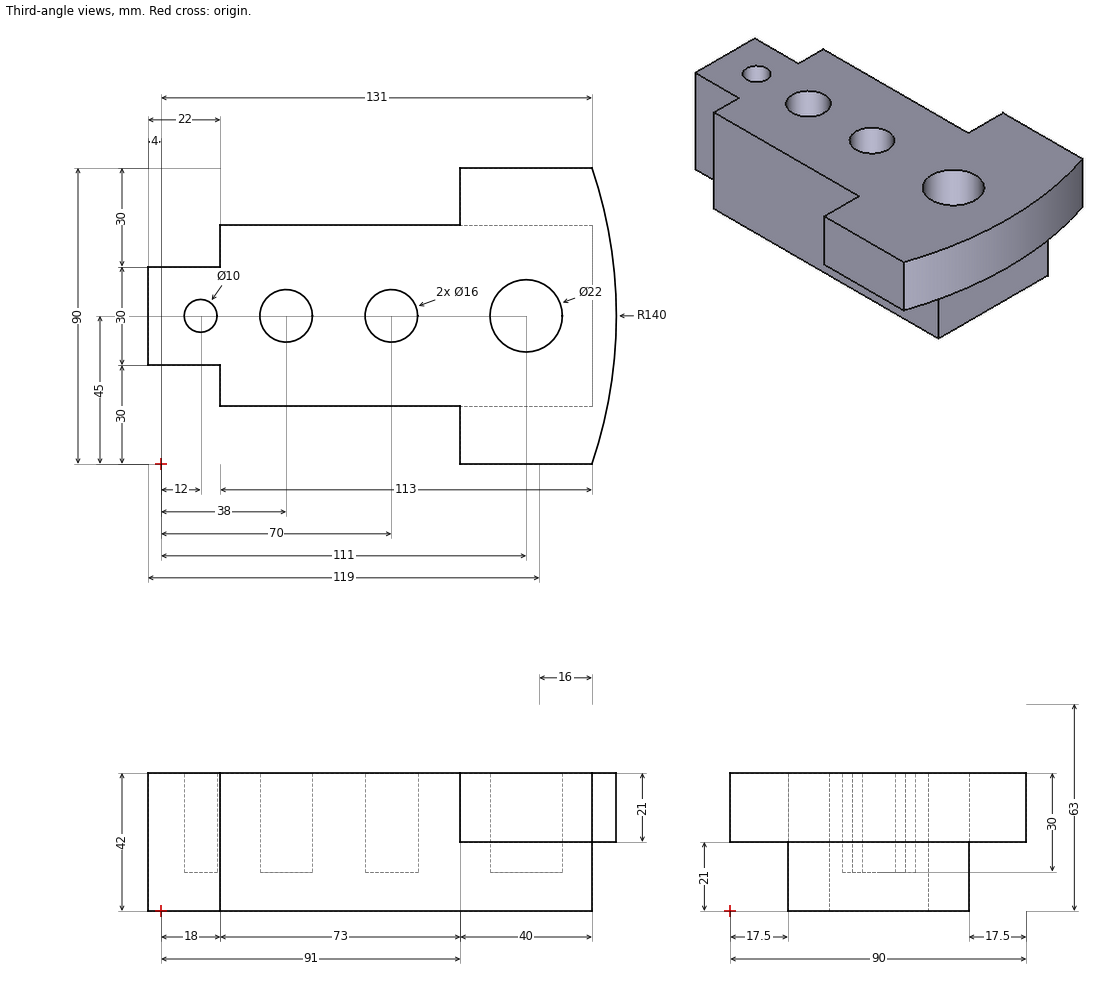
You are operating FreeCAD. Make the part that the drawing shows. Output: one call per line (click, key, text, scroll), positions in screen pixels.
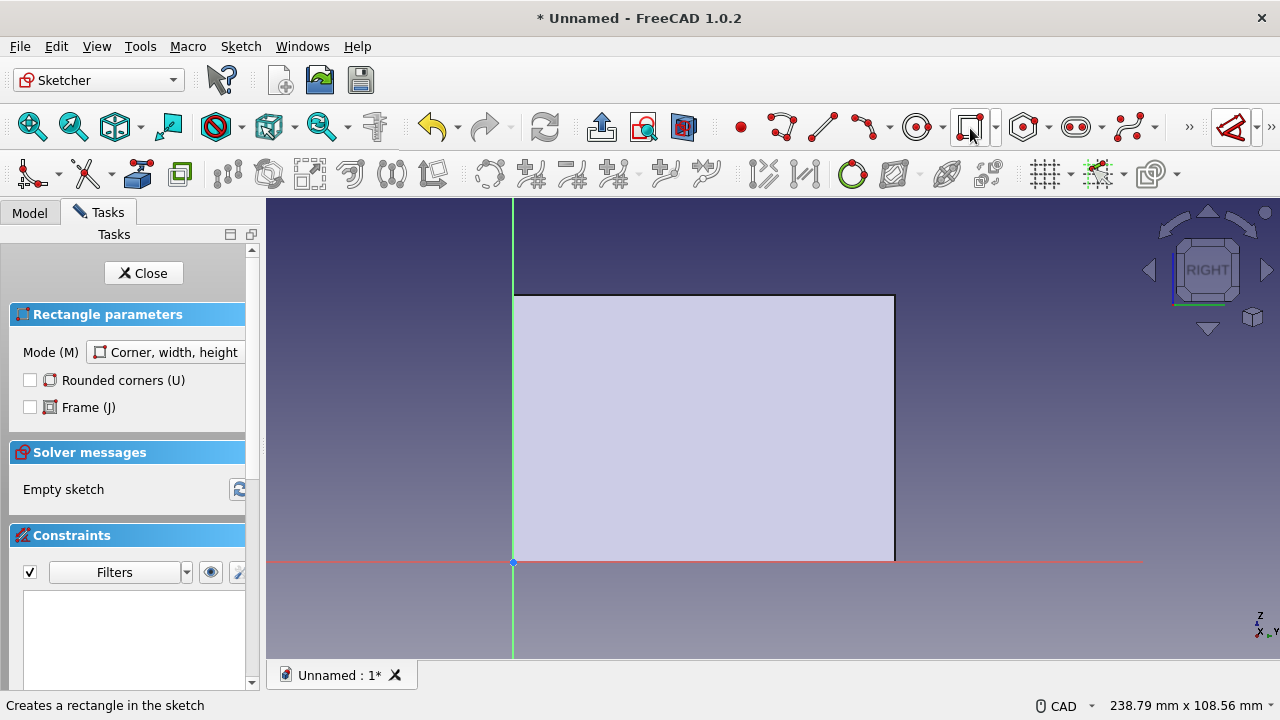
click(513, 562)
move(895, 295)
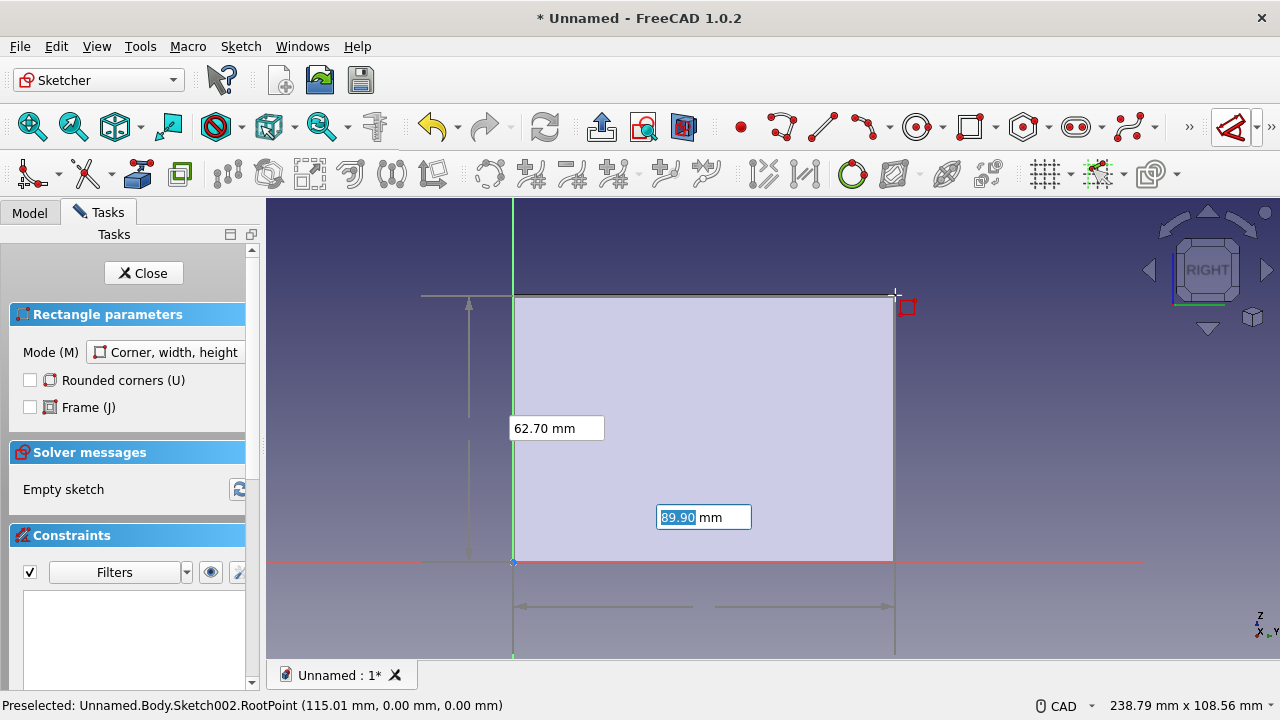
text(90)
key(Tab)
text(63)
key(Return)
key(Escape)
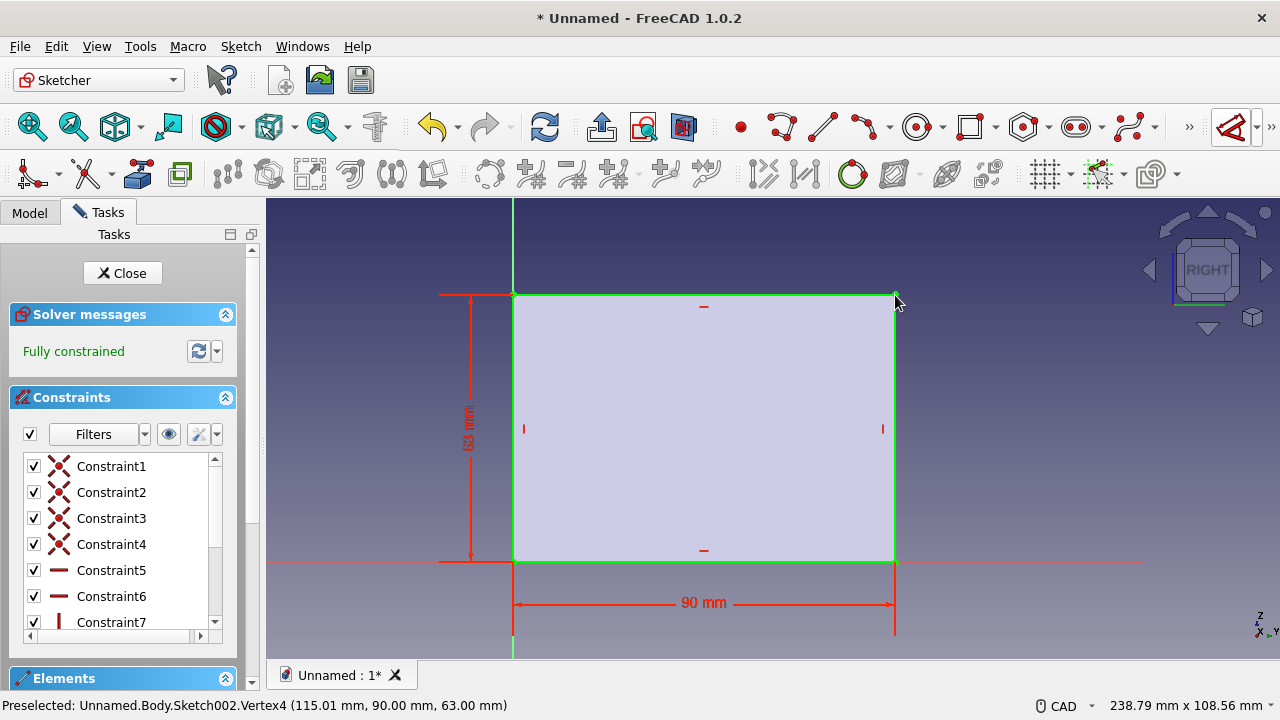
click(123, 273)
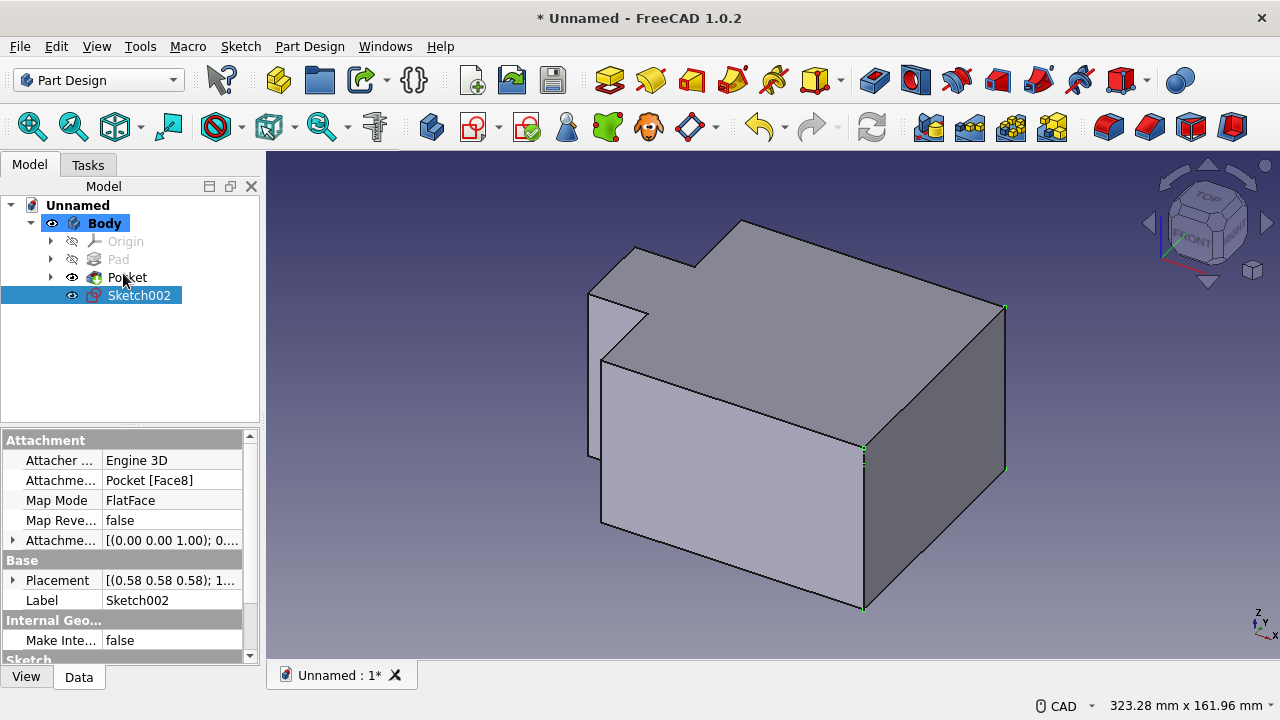
click(610, 80)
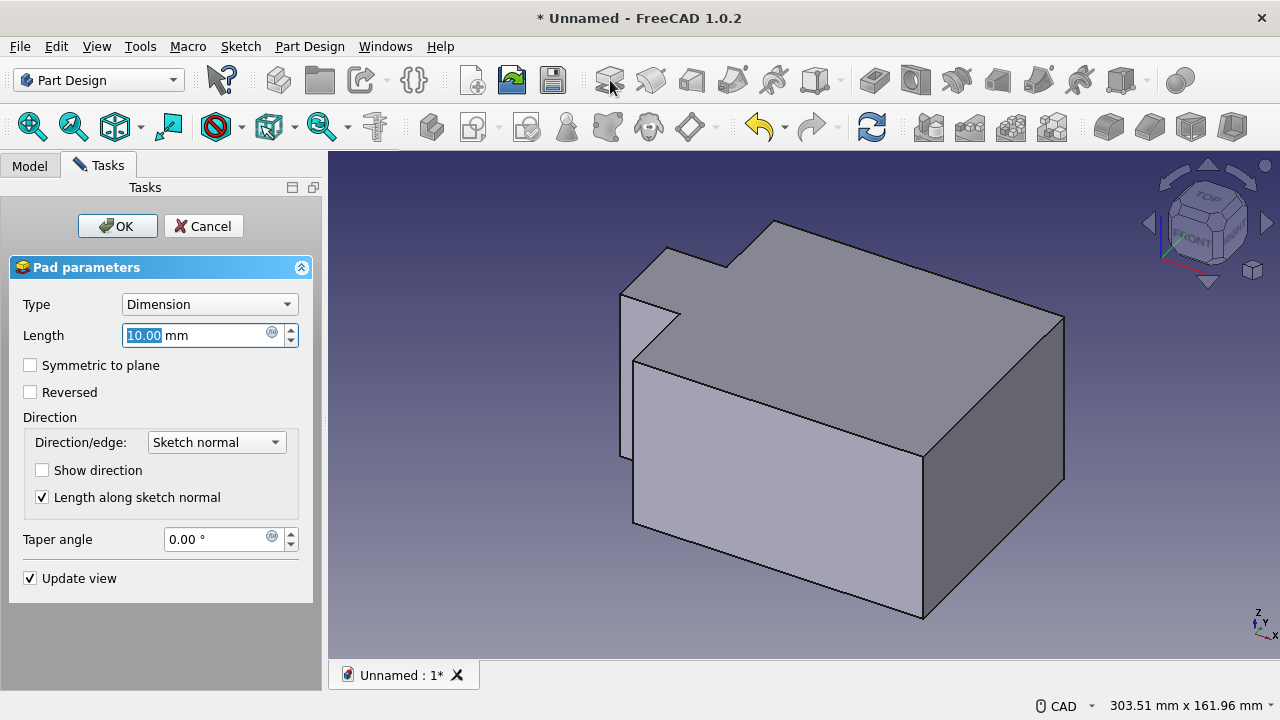
text(16)
key(Tab)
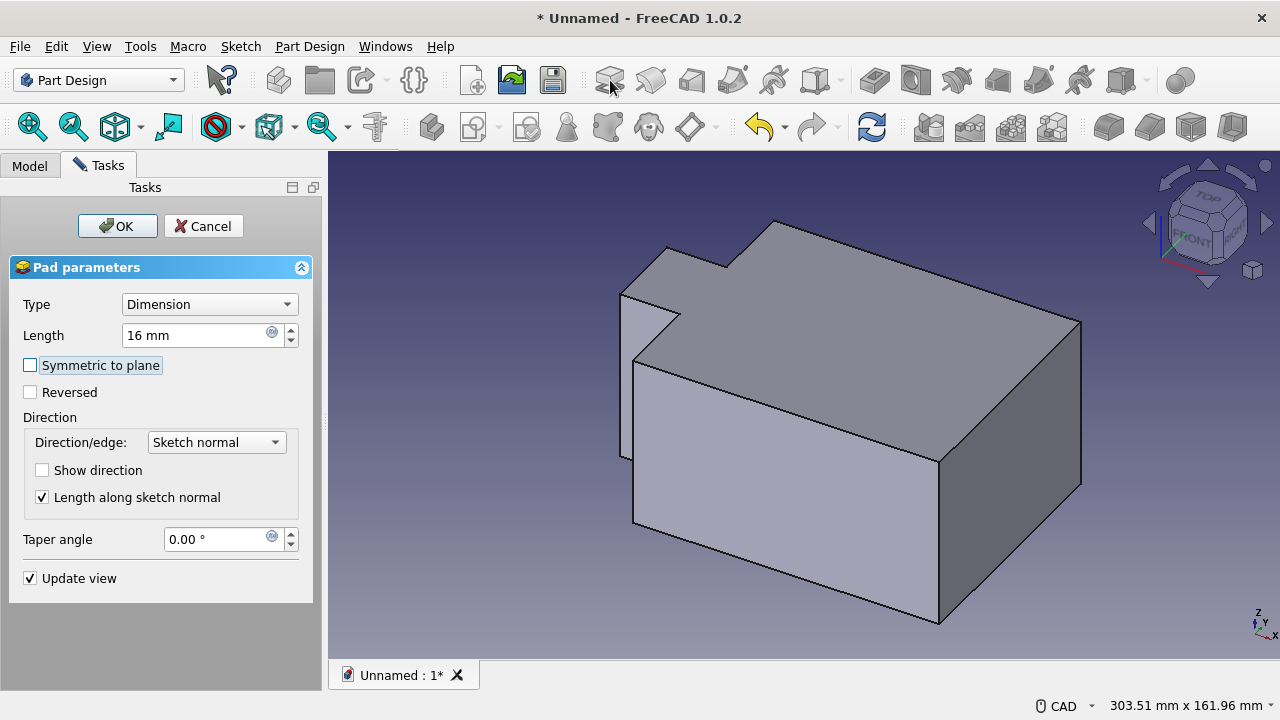
click(118, 226)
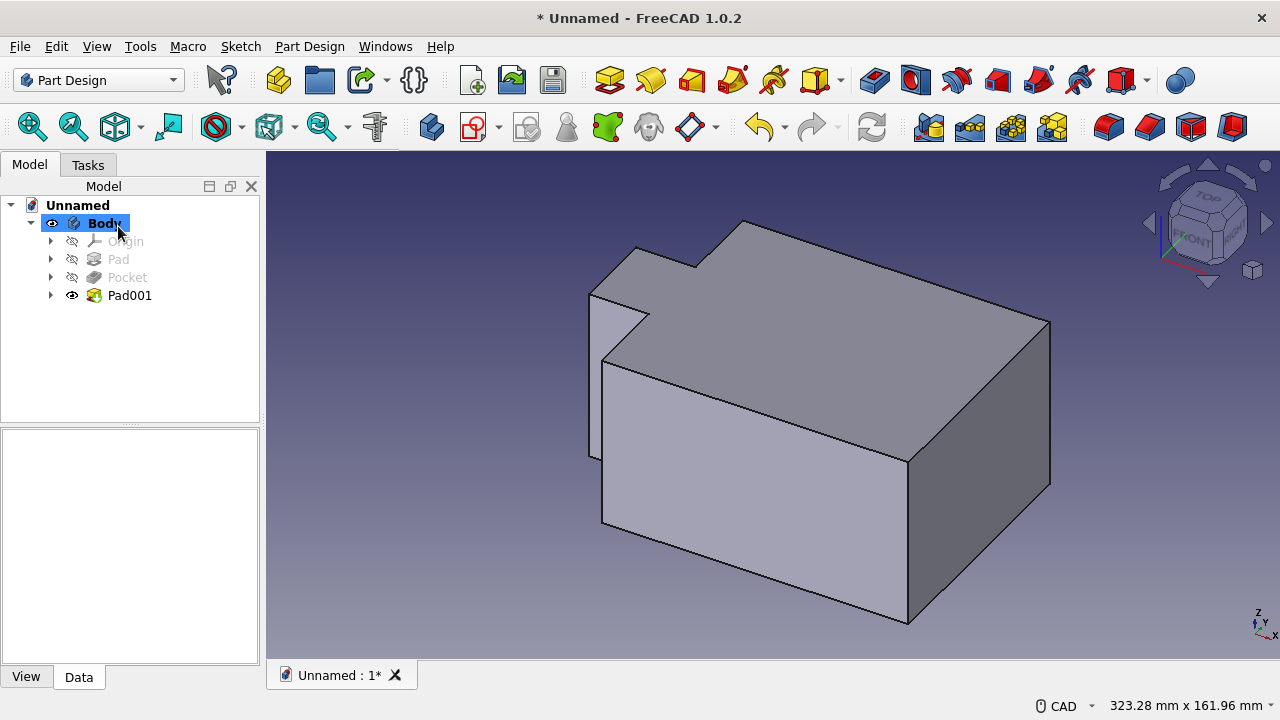
click(848, 348)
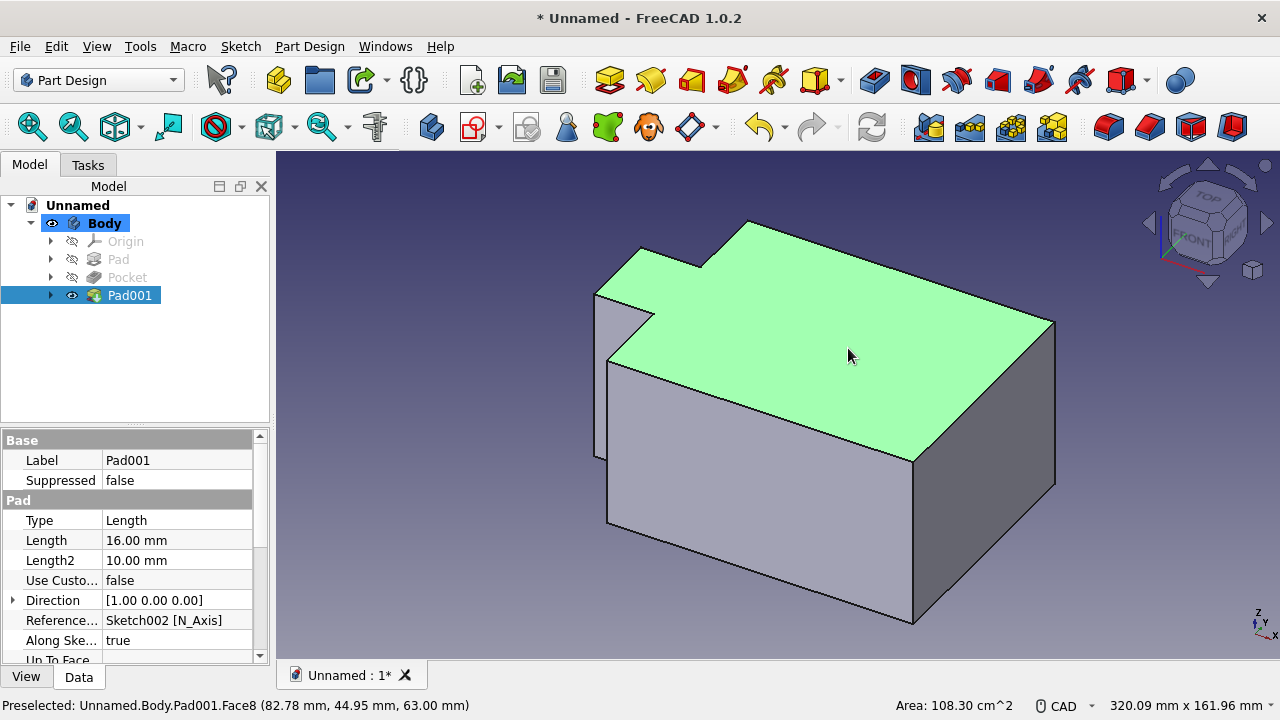
click(472, 128)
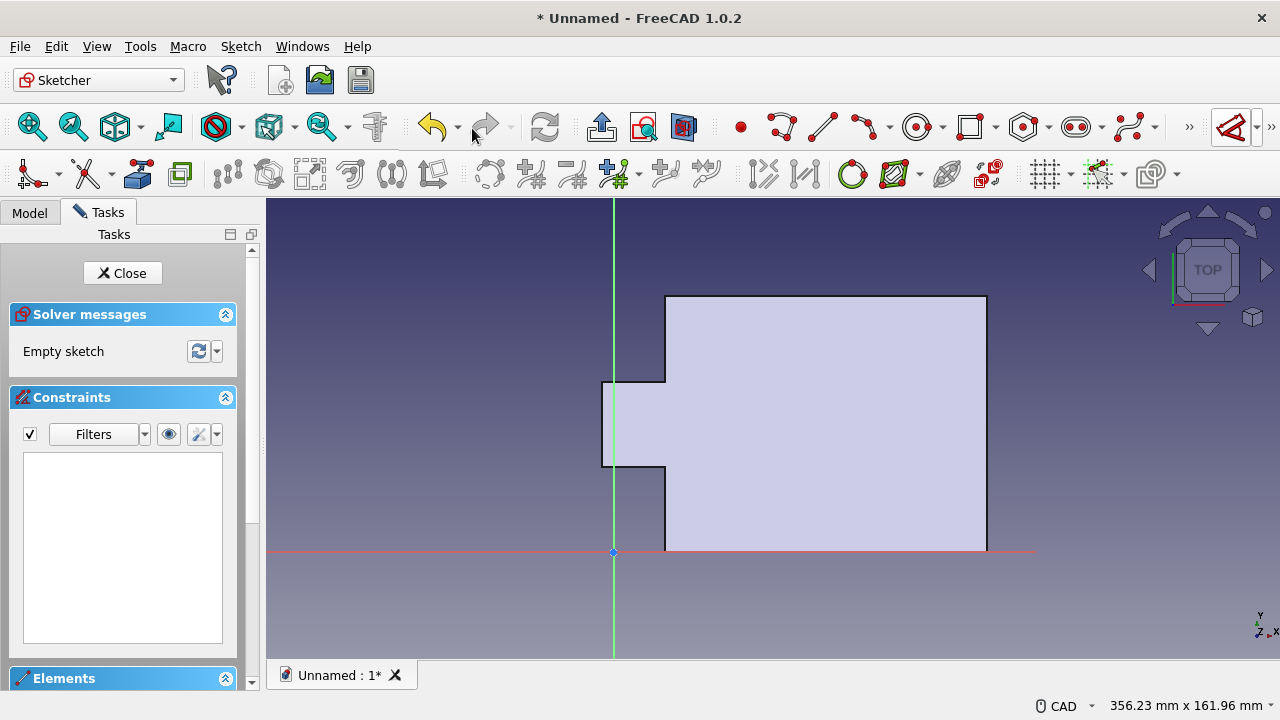
click(782, 128)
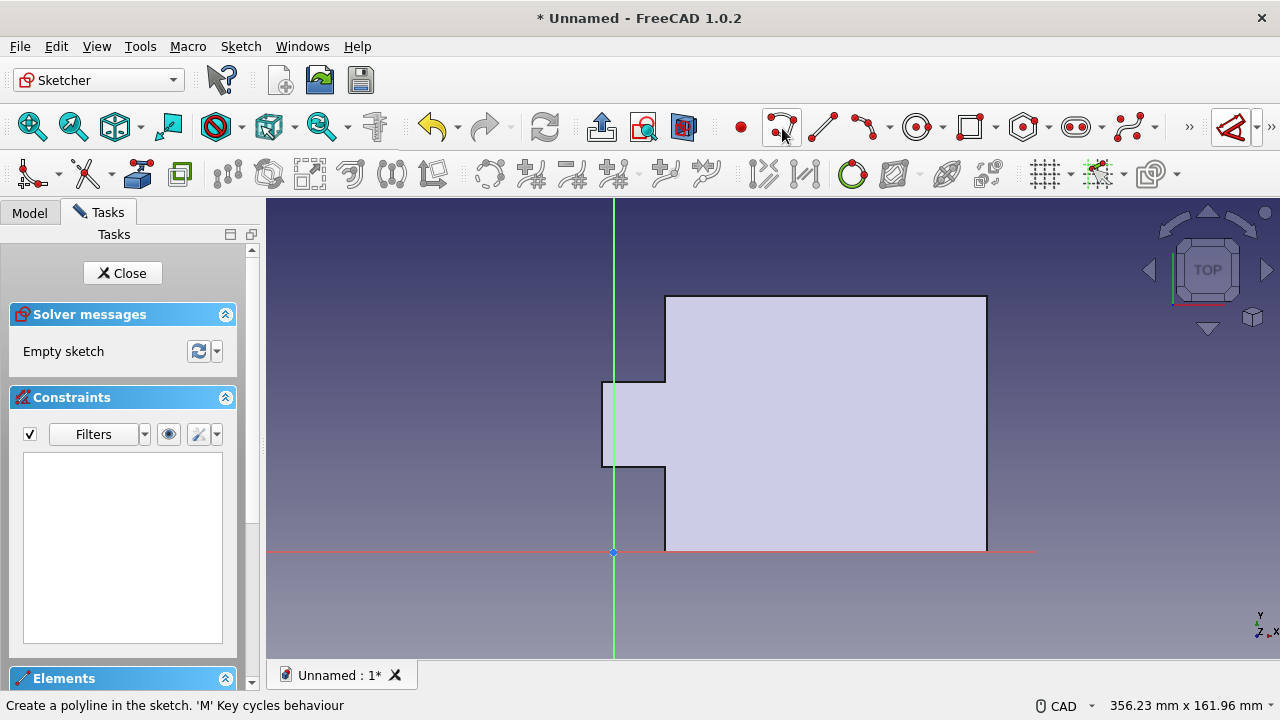
click(665, 552)
click(987, 543)
click(987, 296)
click(665, 296)
click(665, 382)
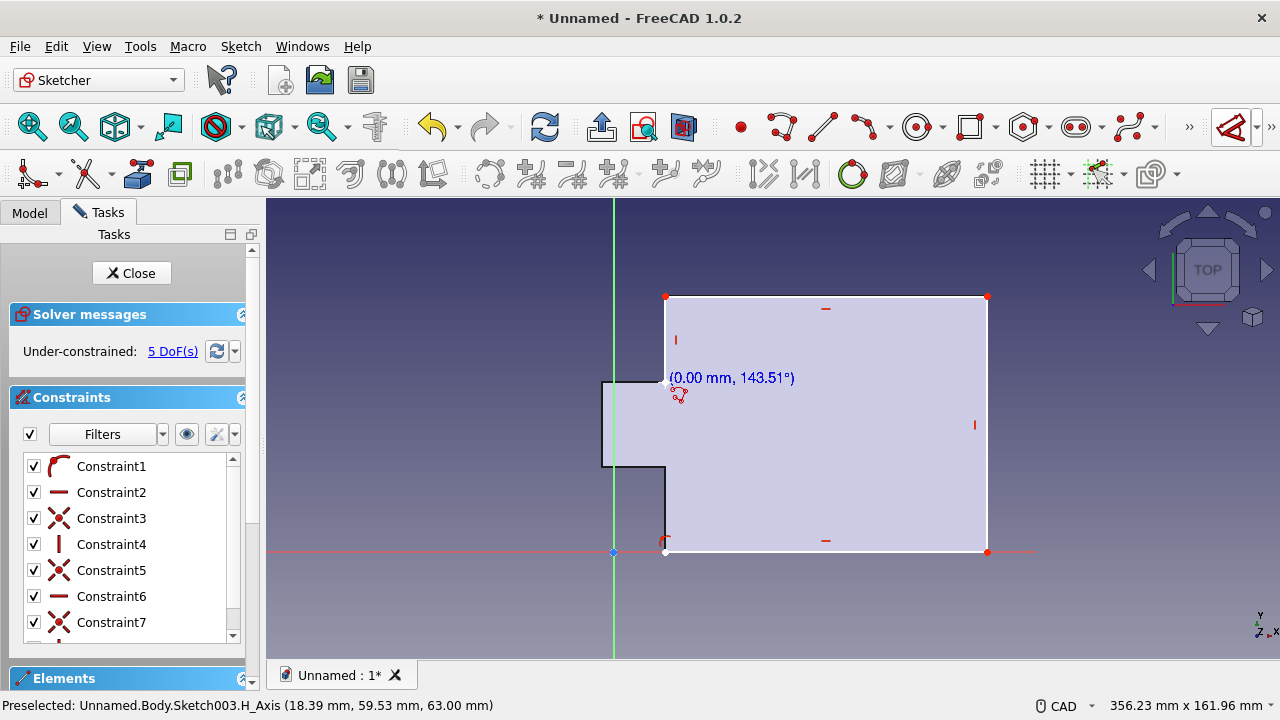
scroll(602, 382, up, 2)